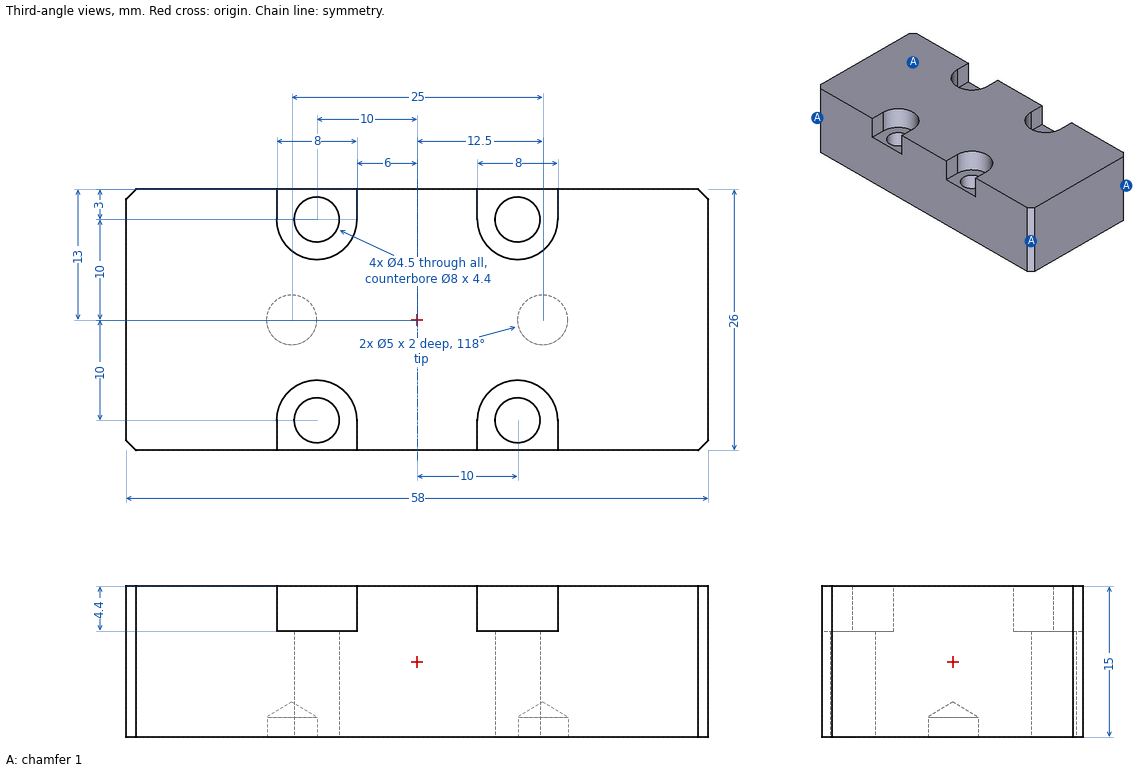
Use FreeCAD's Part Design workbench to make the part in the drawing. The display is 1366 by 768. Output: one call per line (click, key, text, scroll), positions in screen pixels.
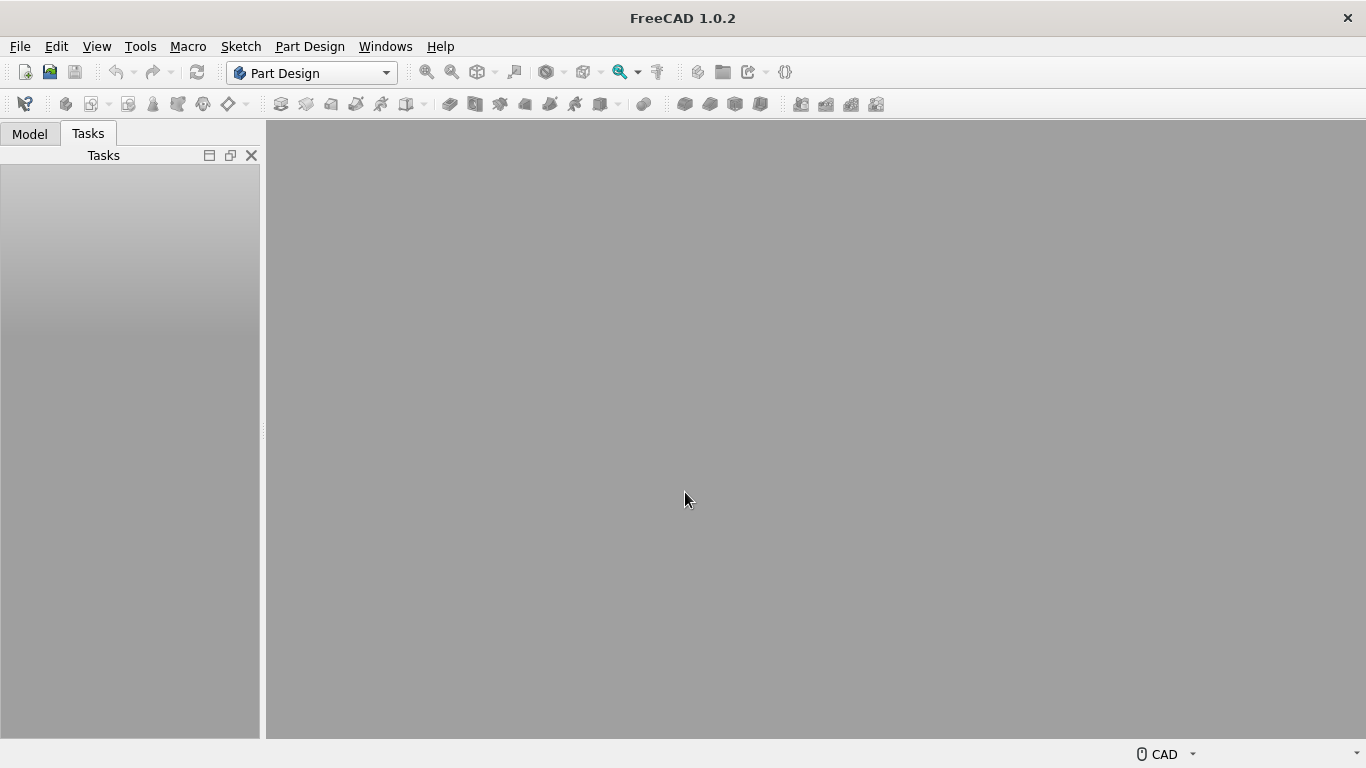
click(25, 72)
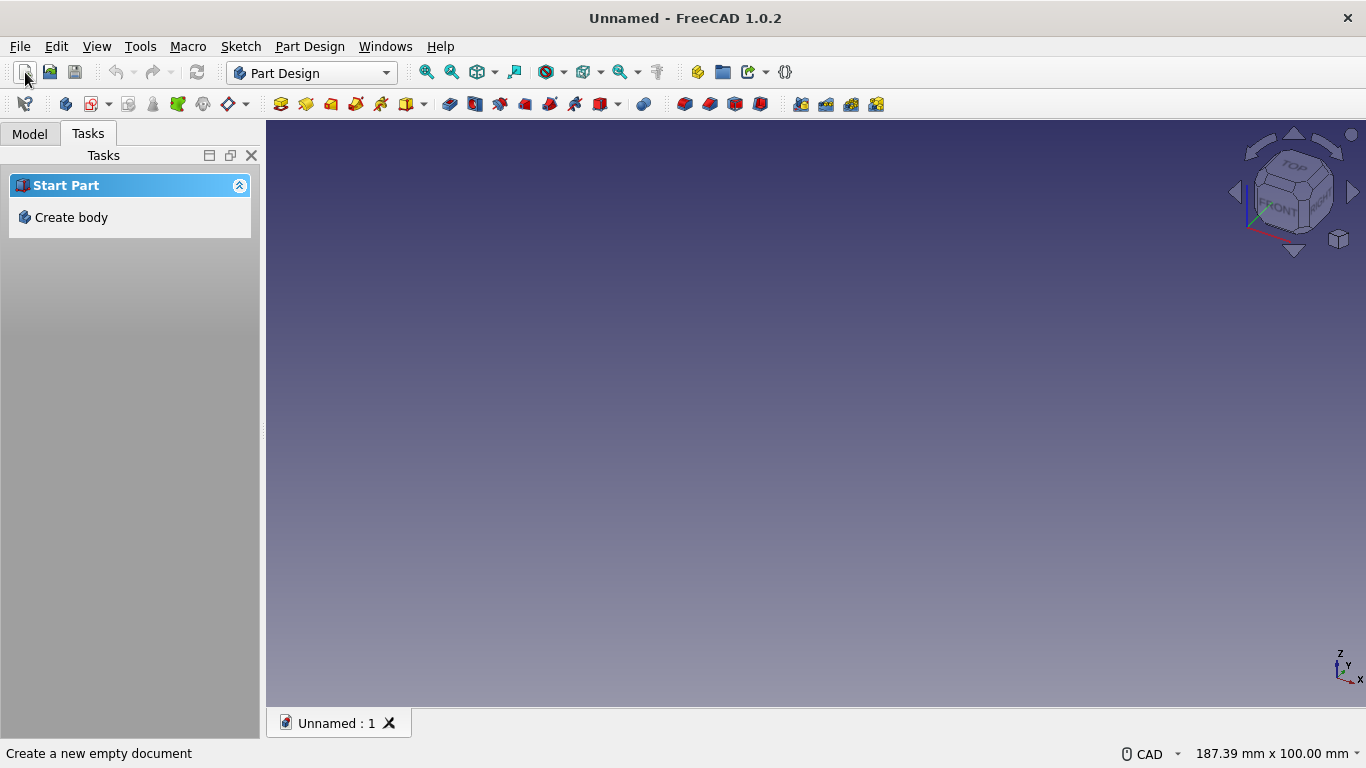
click(90, 104)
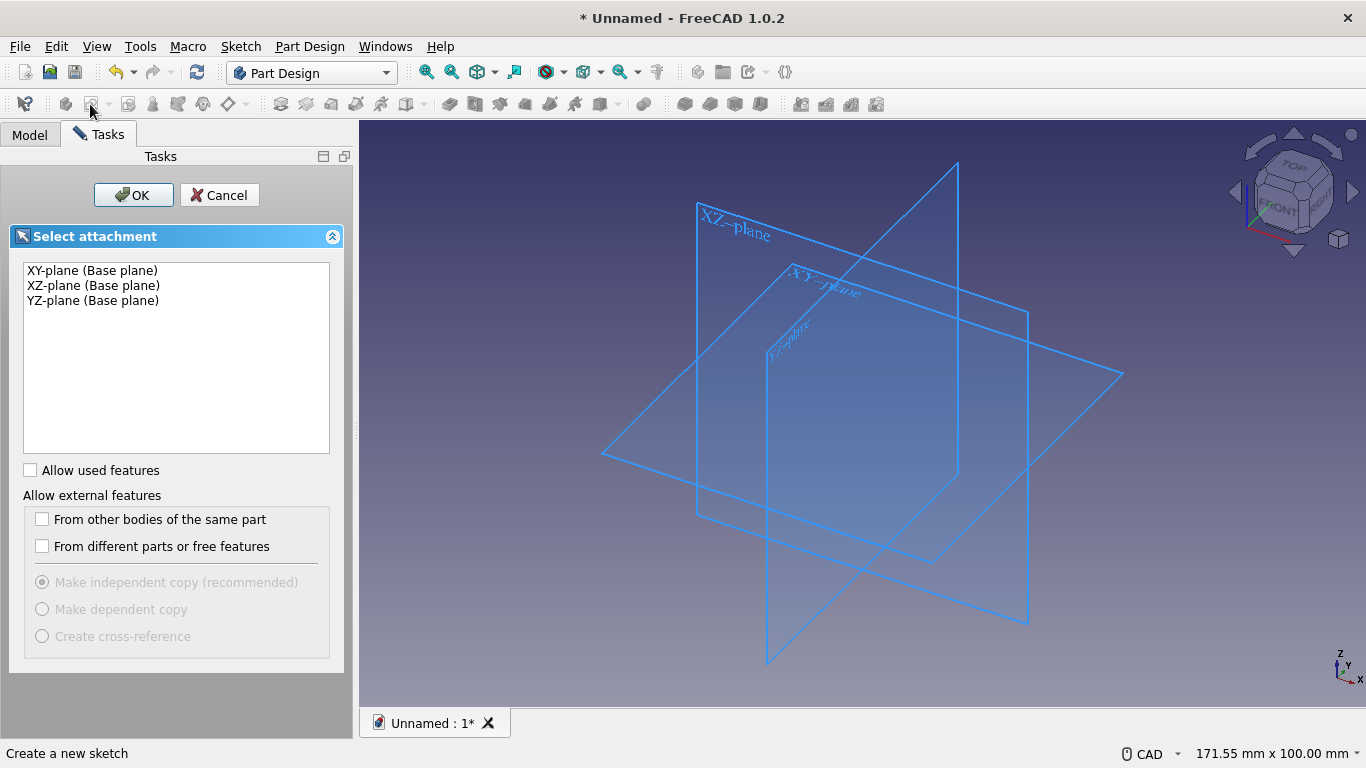
click(84, 270)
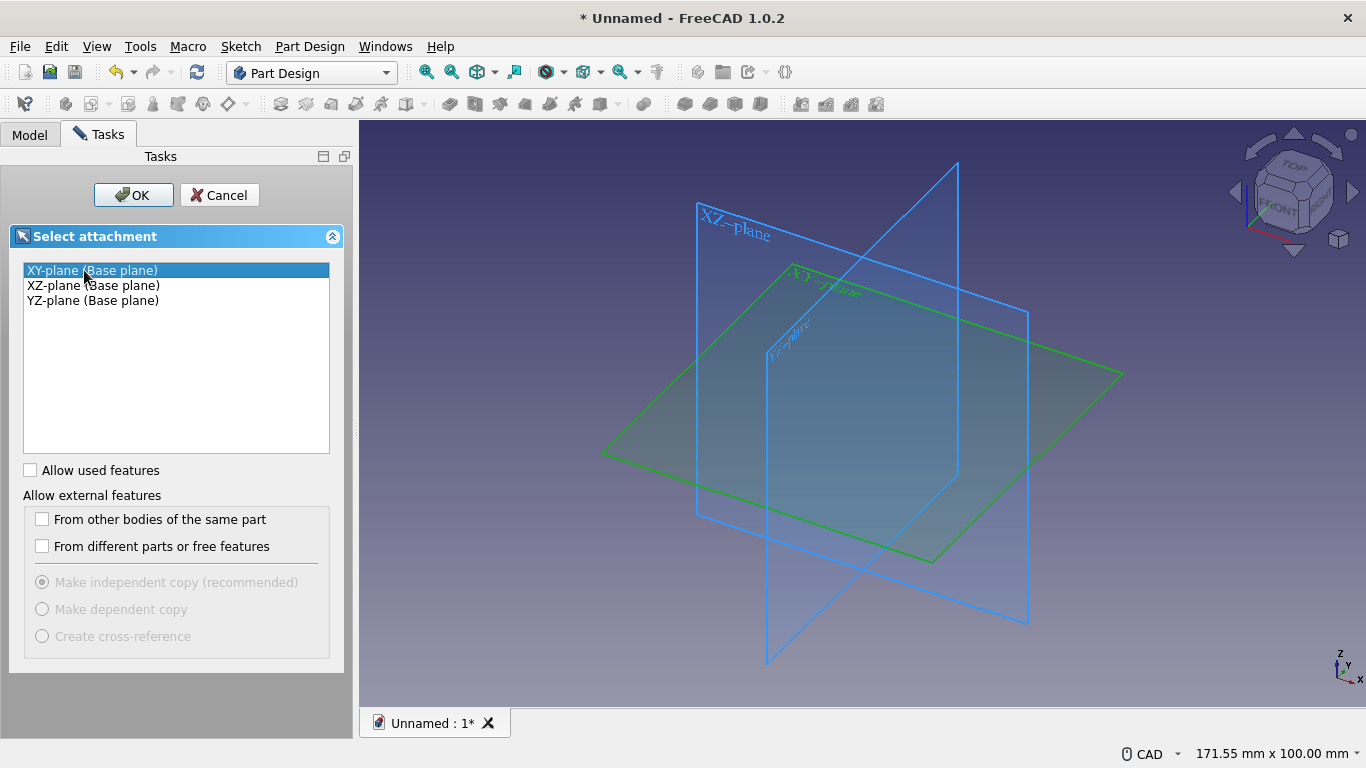
click(134, 195)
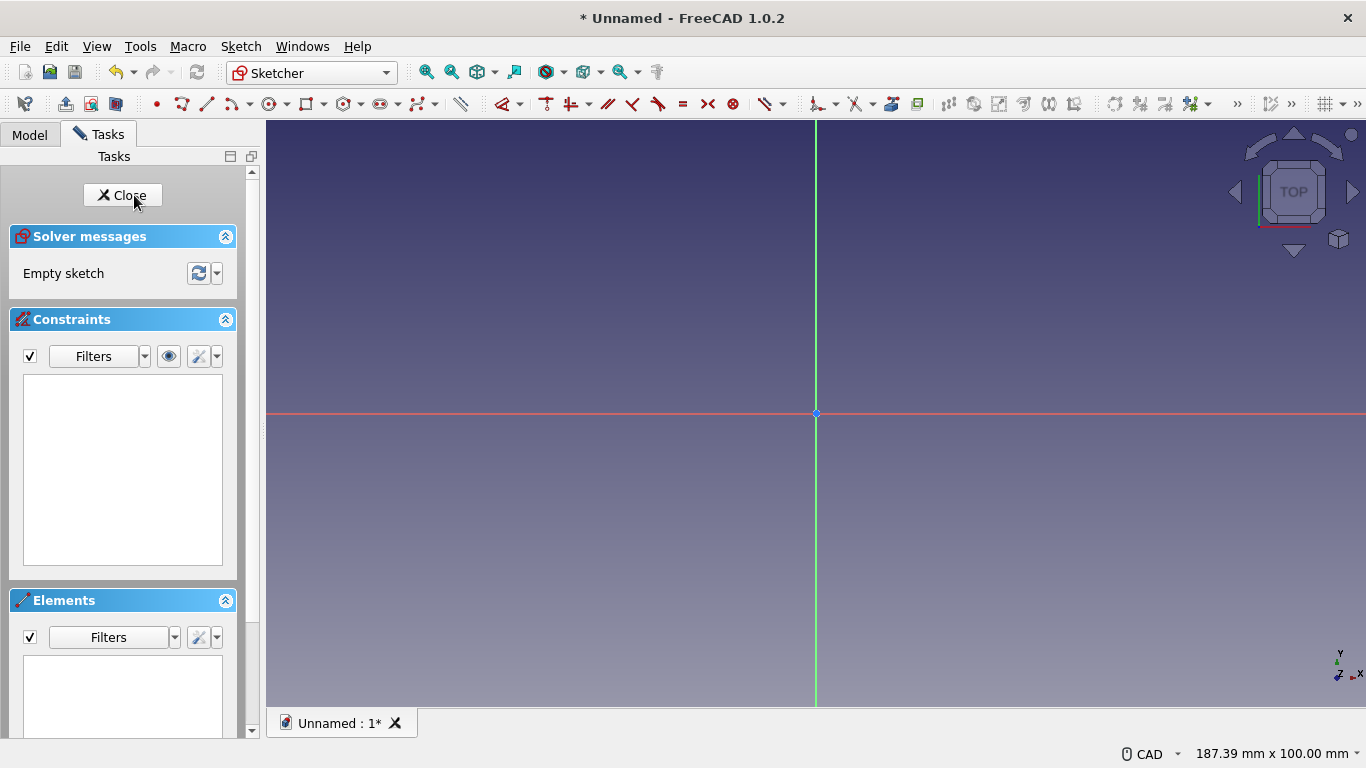
scroll(899, 414, up, 3)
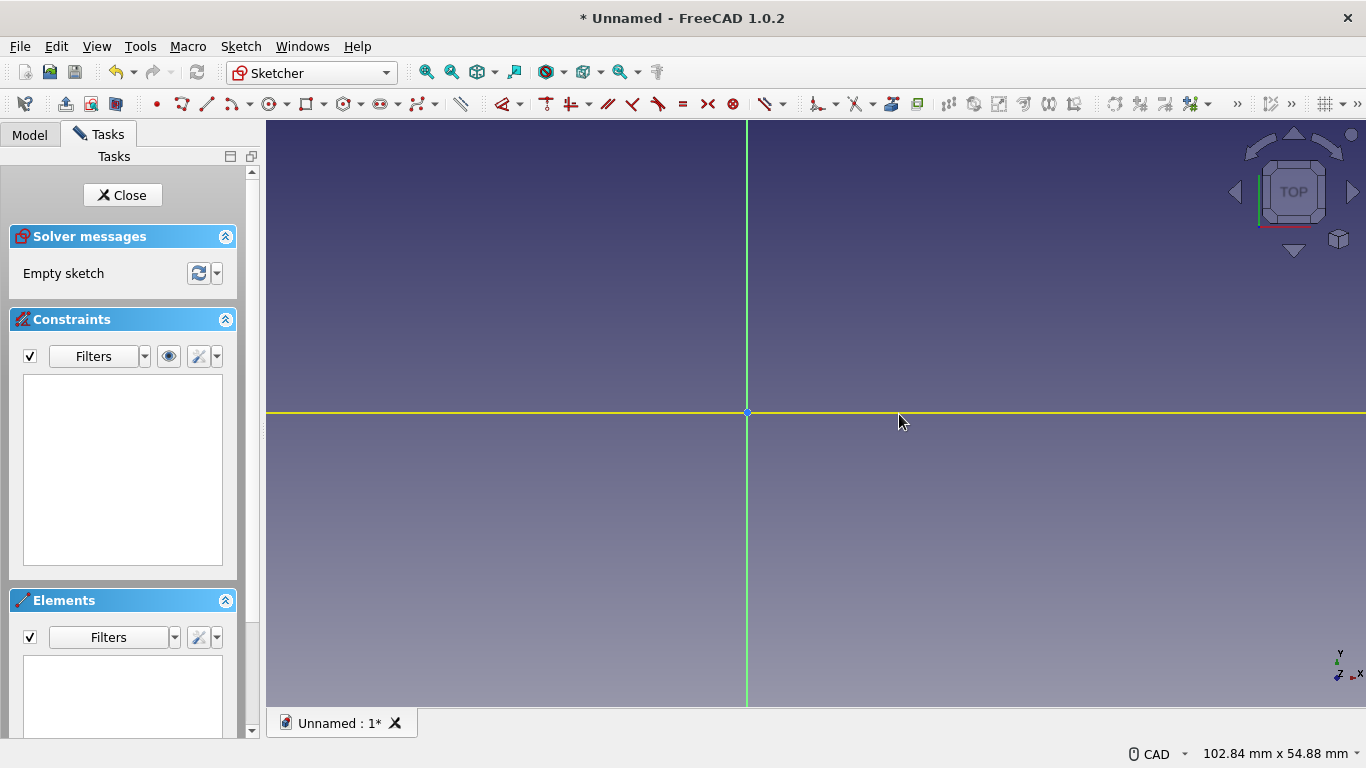
key(g)
key(v)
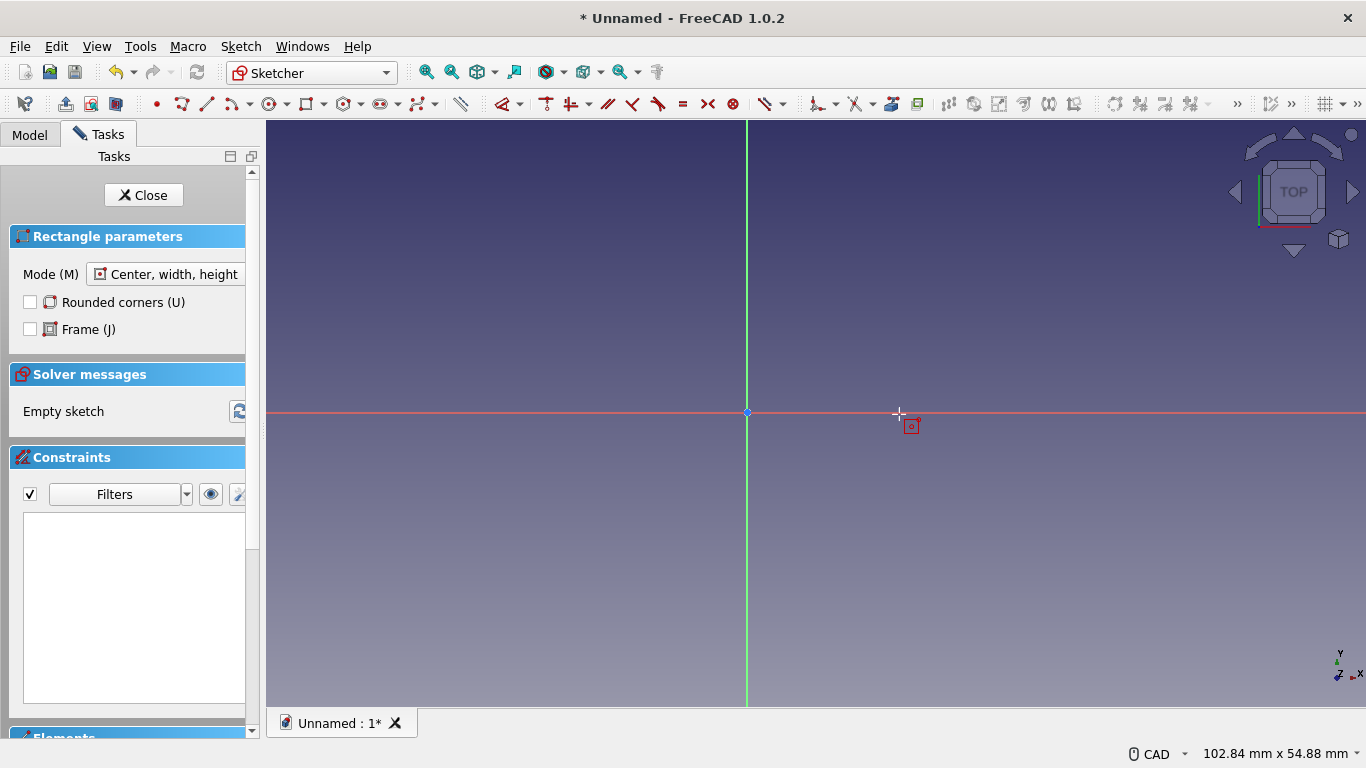
click(747, 413)
move(1057, 274)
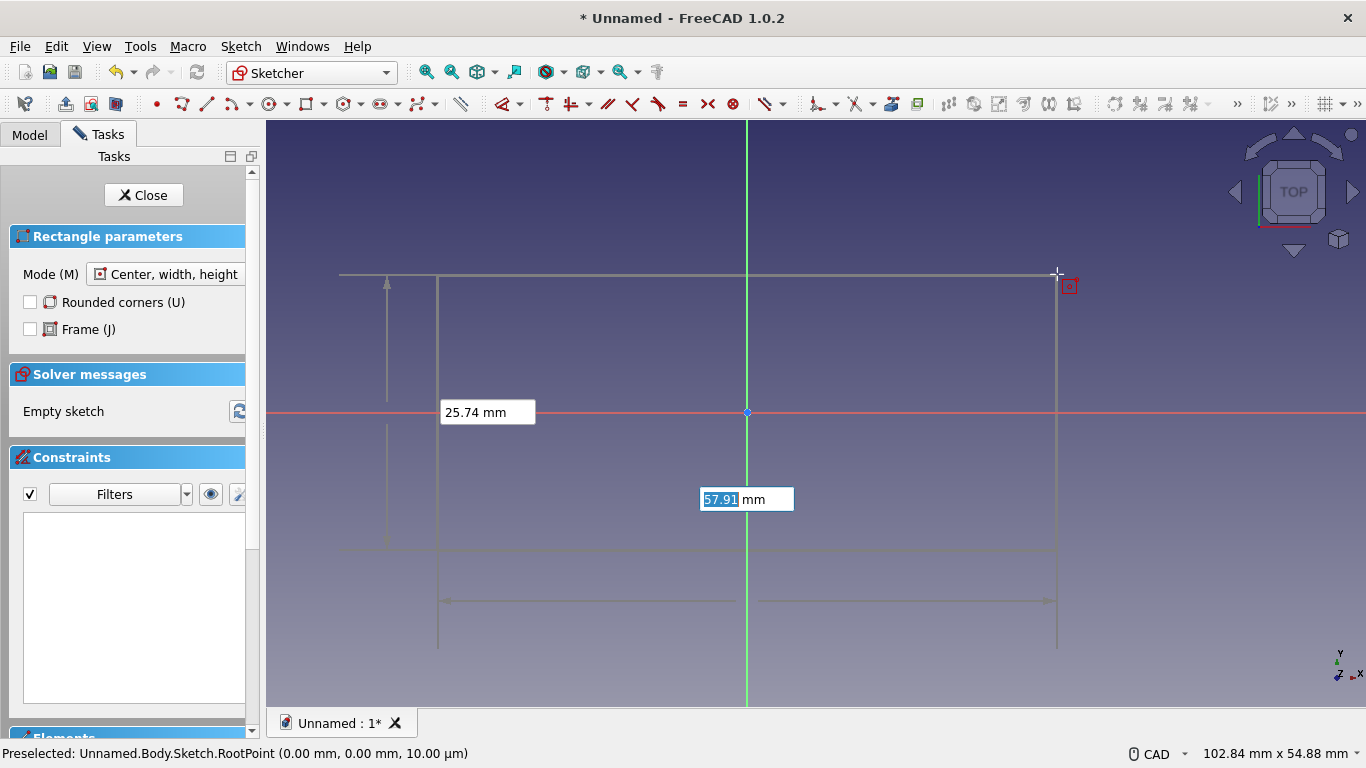
text(58)
key(Tab)
text(26)
key(Return)
key(Escape)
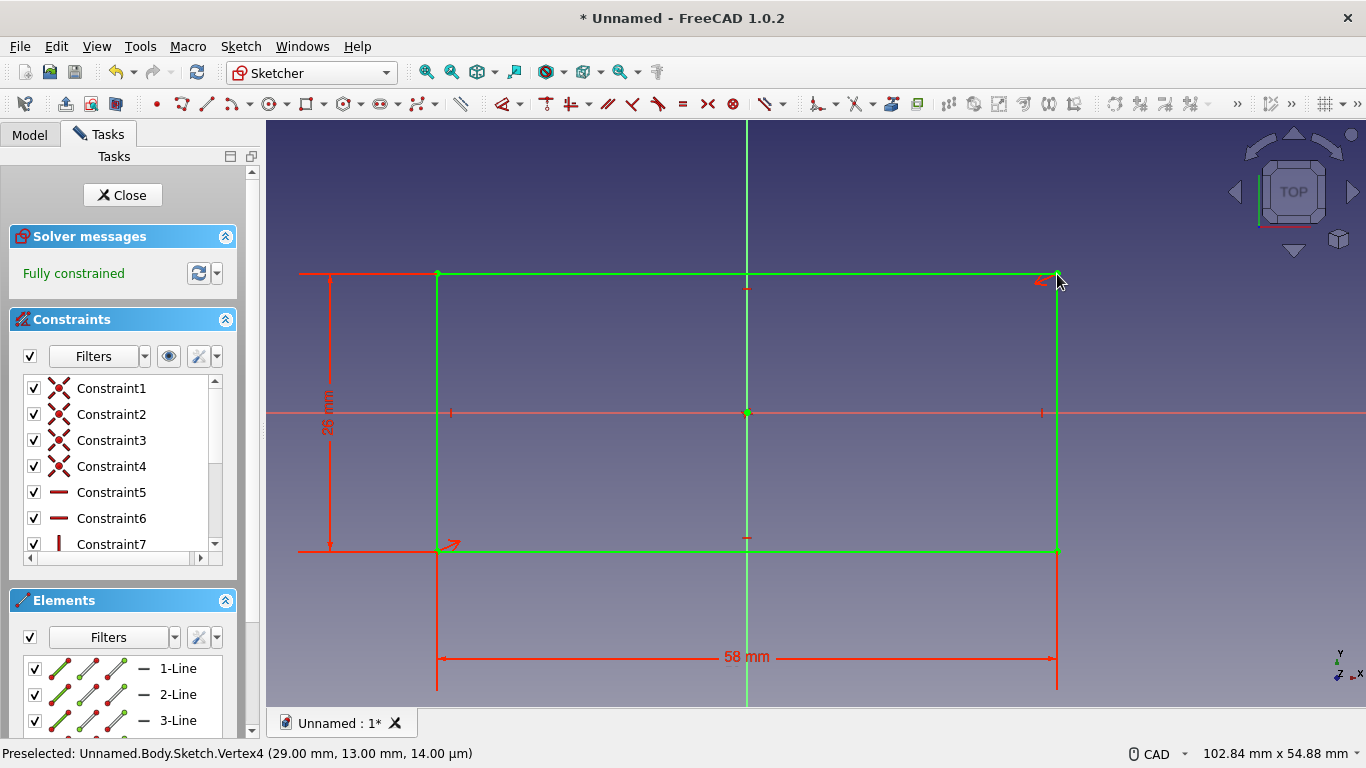
click(123, 195)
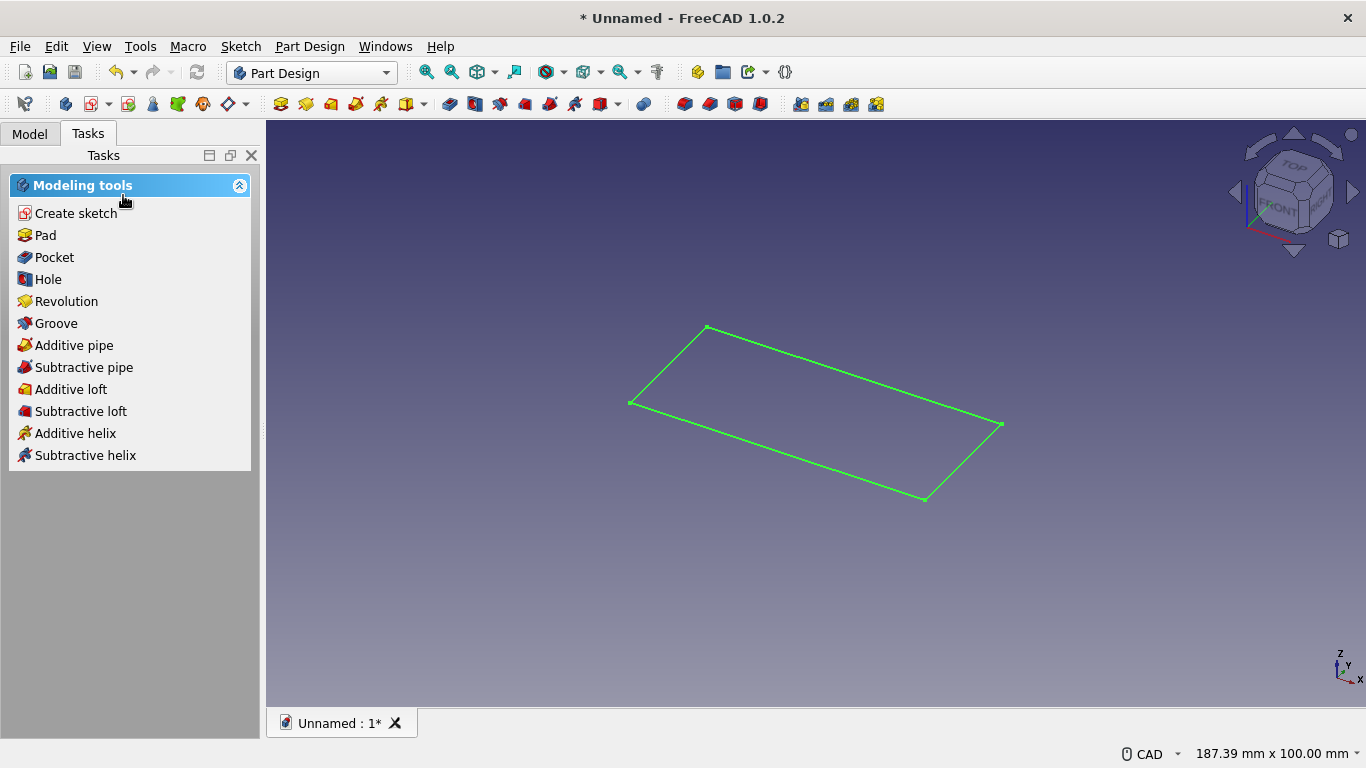
click(281, 104)